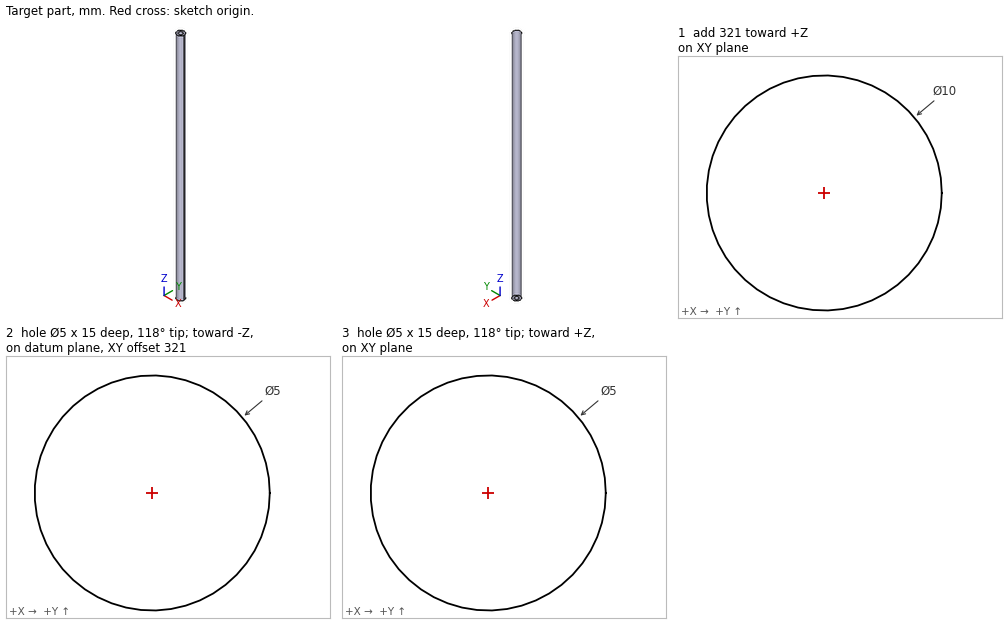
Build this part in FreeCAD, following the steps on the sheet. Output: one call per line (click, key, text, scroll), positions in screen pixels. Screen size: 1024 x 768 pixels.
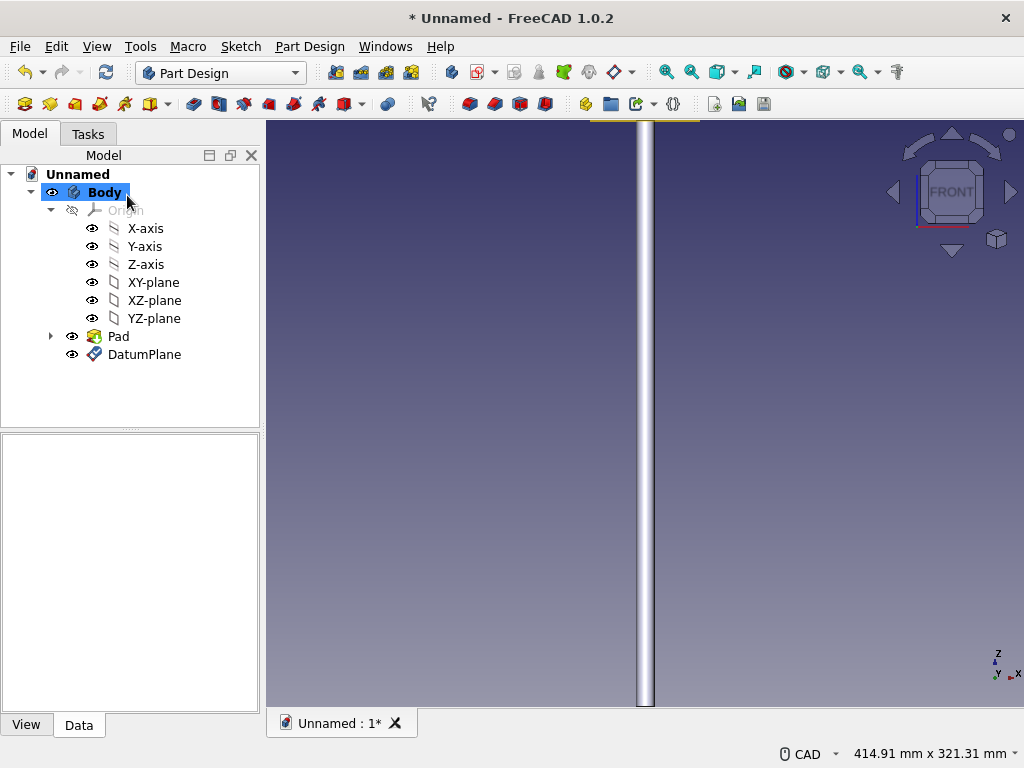
click(117, 354)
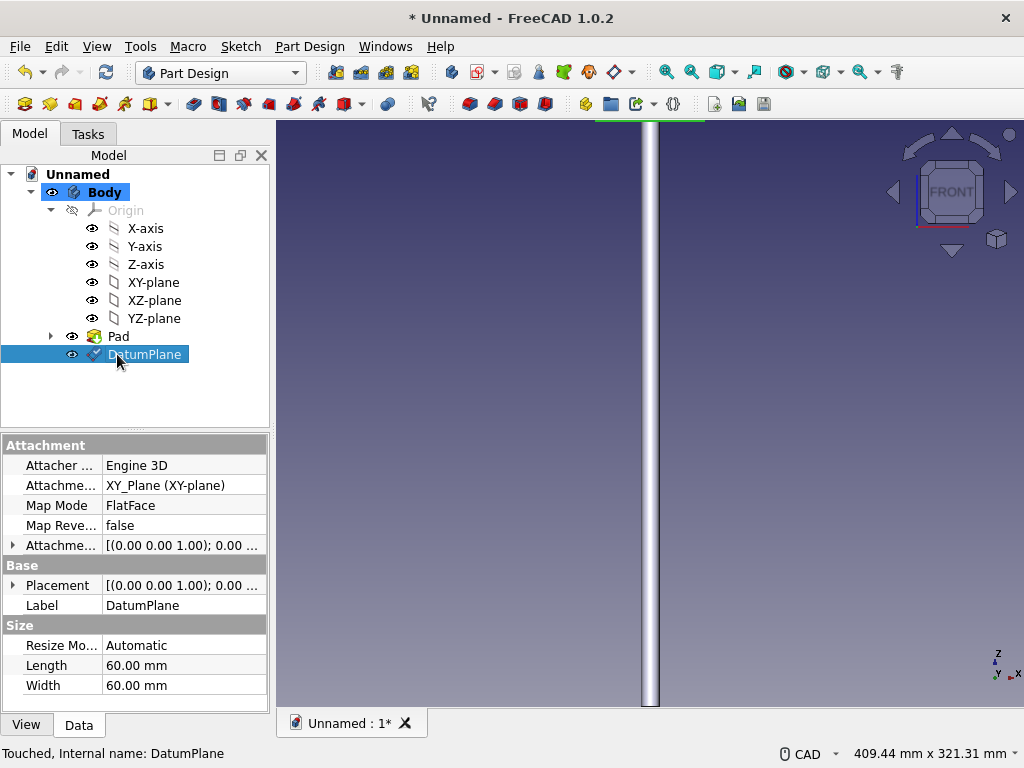
click(476, 72)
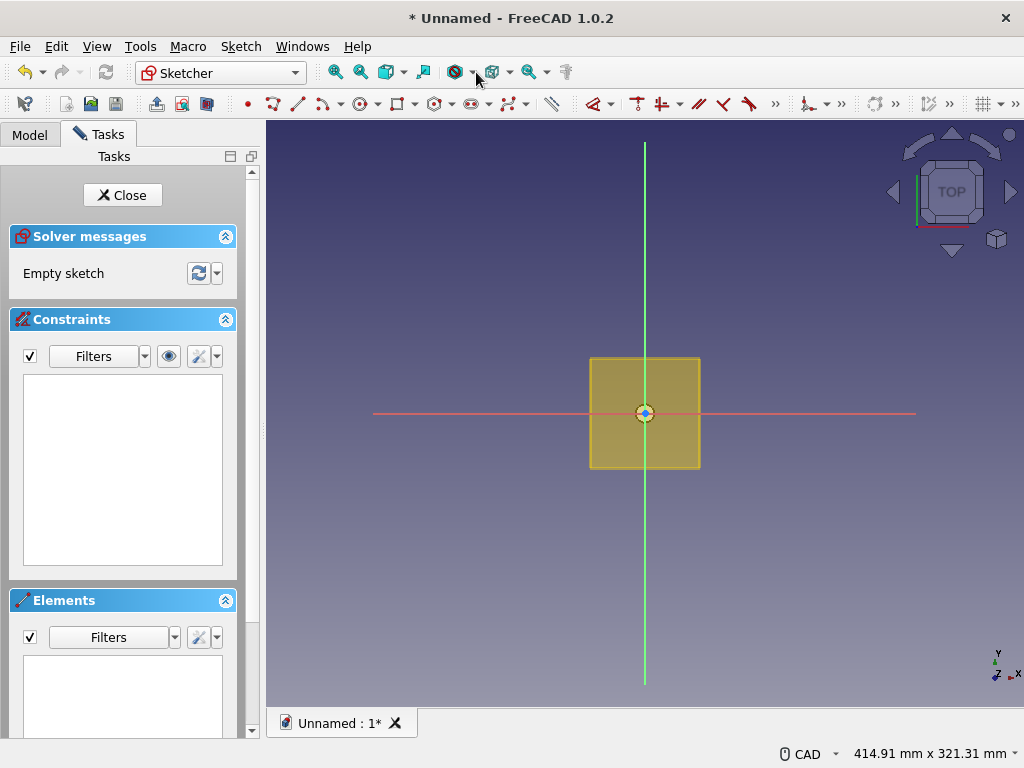
scroll(649, 414, up, 15)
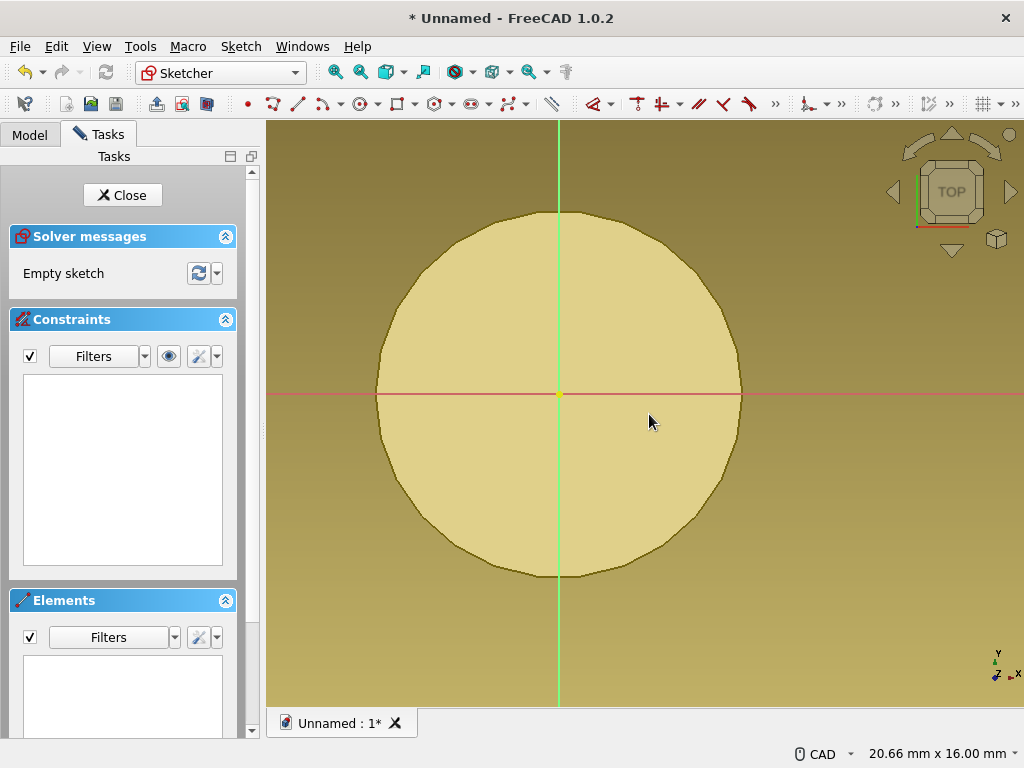
scroll(545, 379, up, 4)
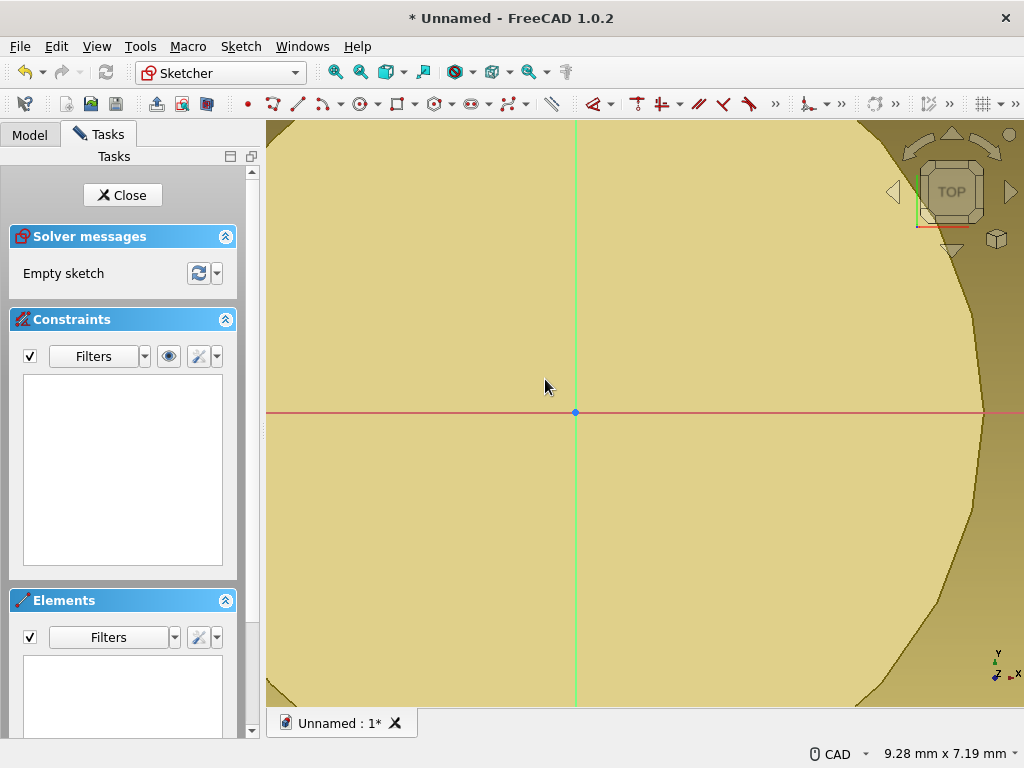
click(360, 104)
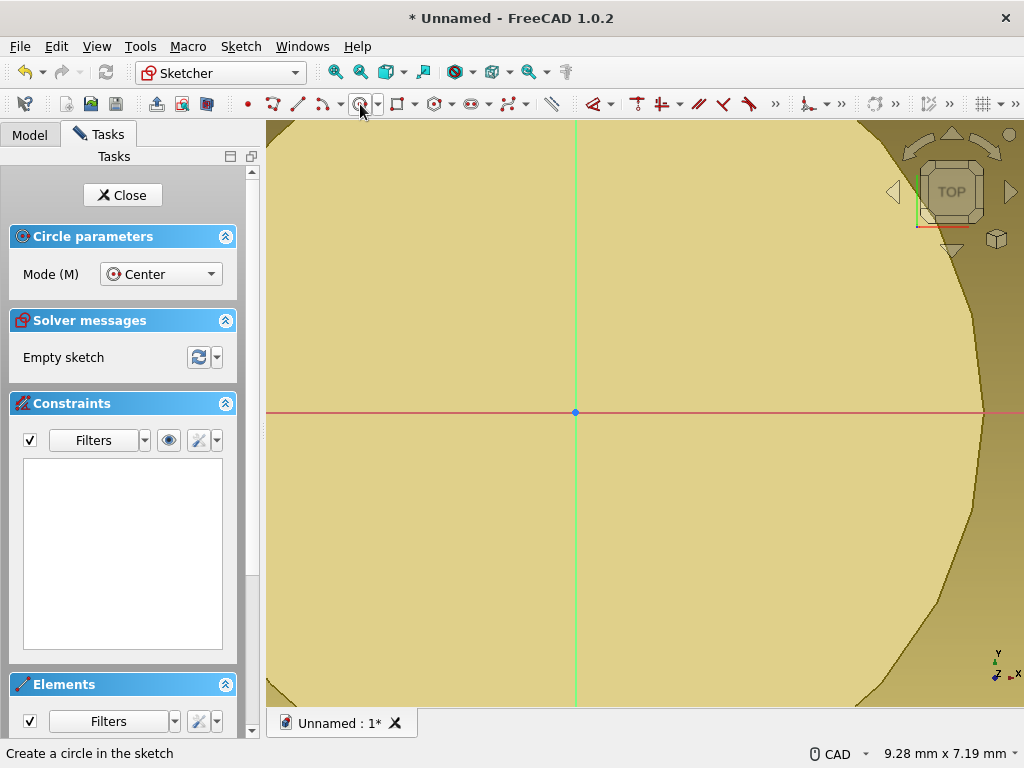
click(576, 413)
move(720, 268)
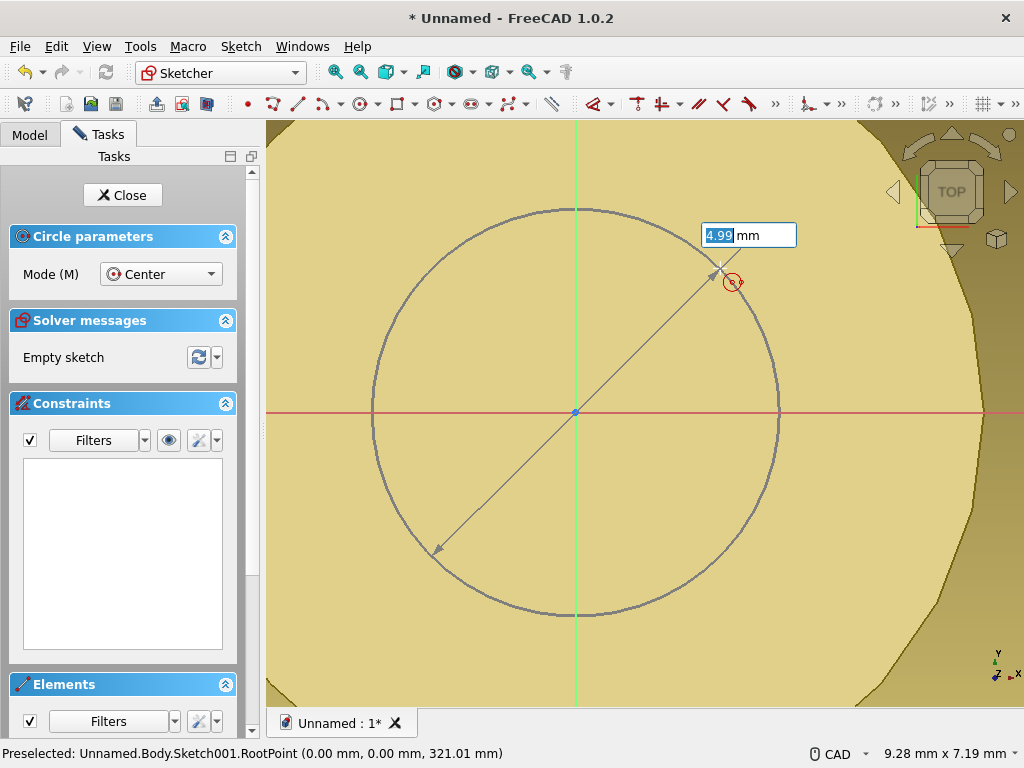
text(5)
key(Return)
key(Escape)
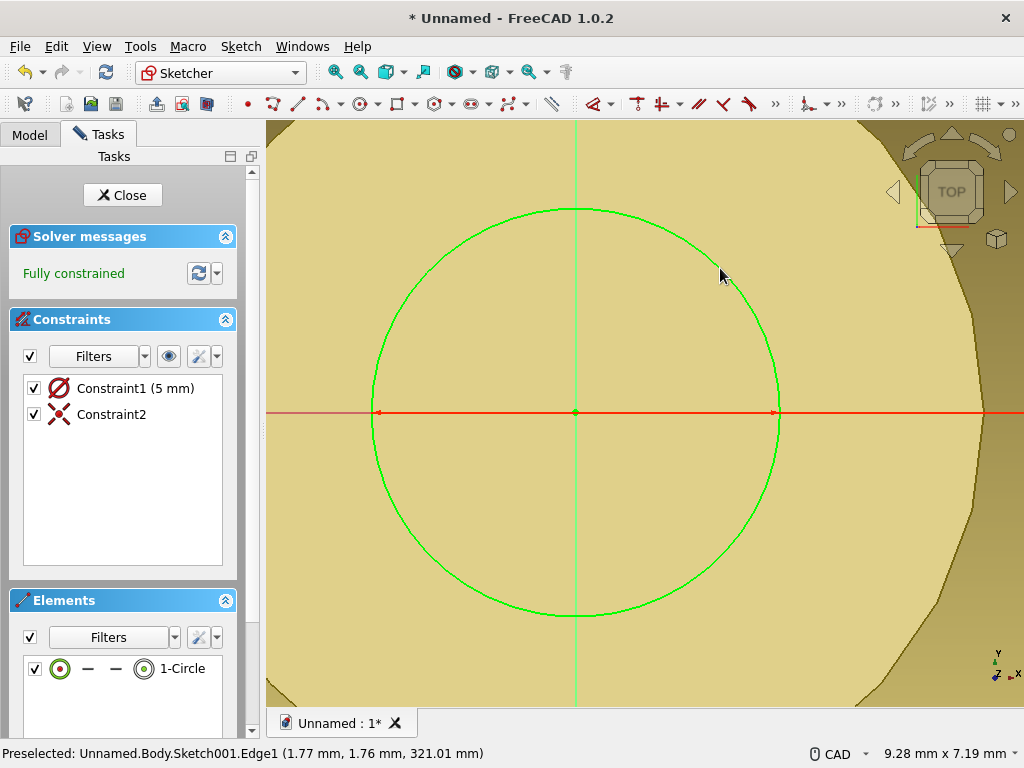
click(123, 195)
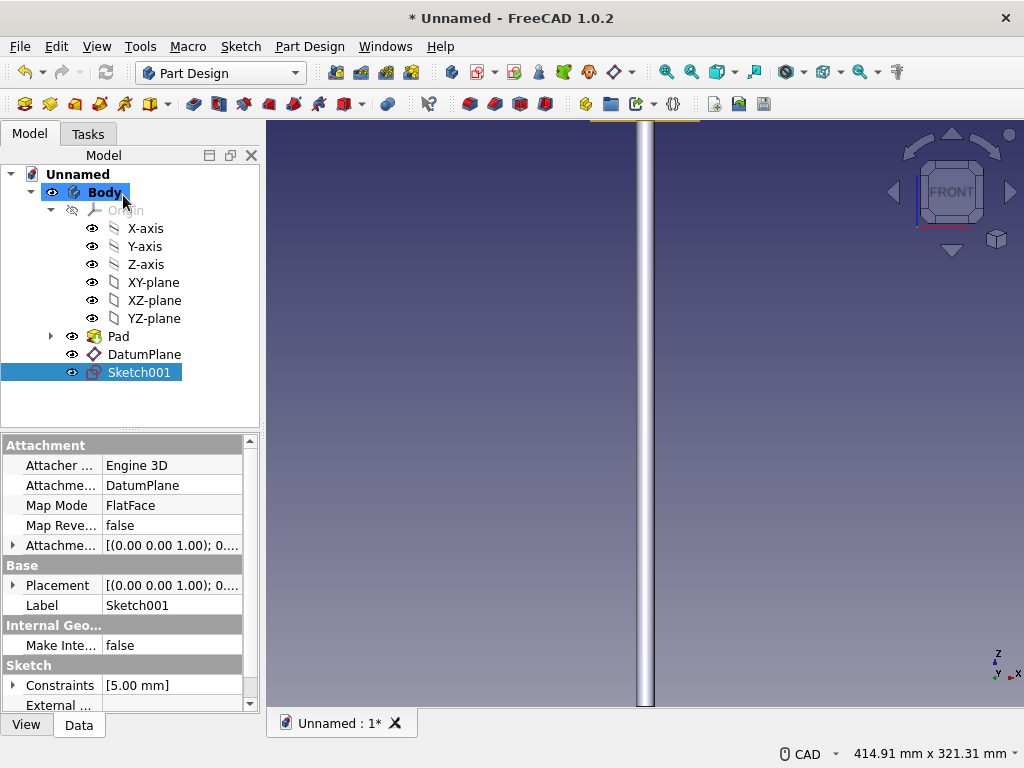
click(219, 104)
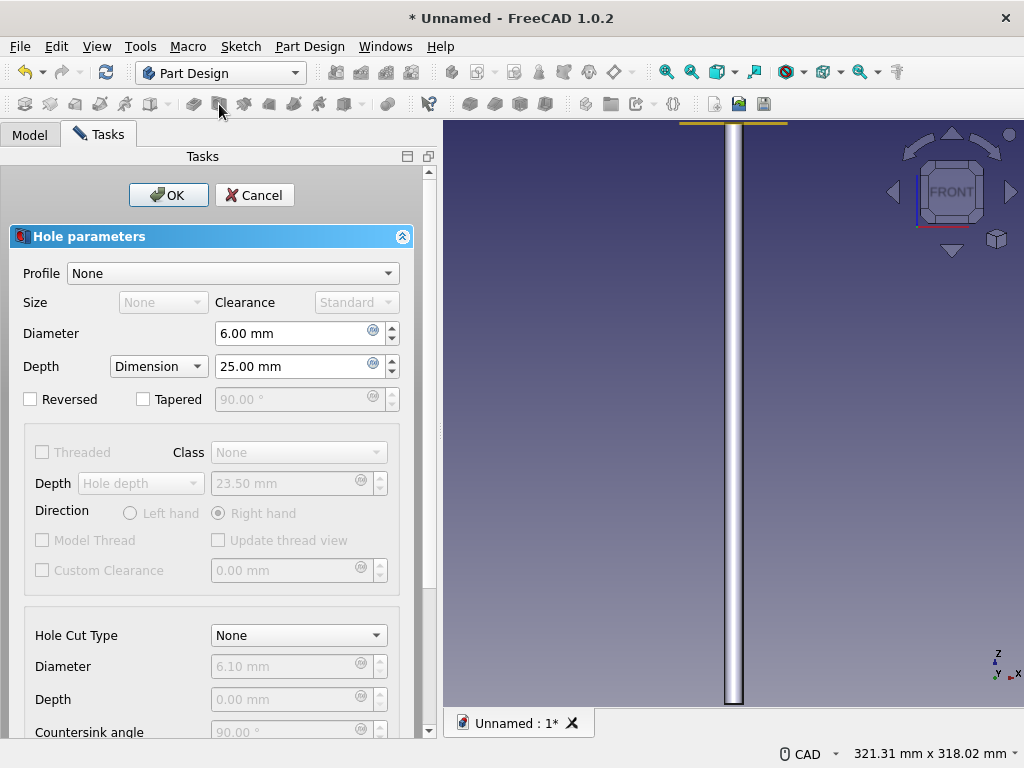
triple_click(300, 334)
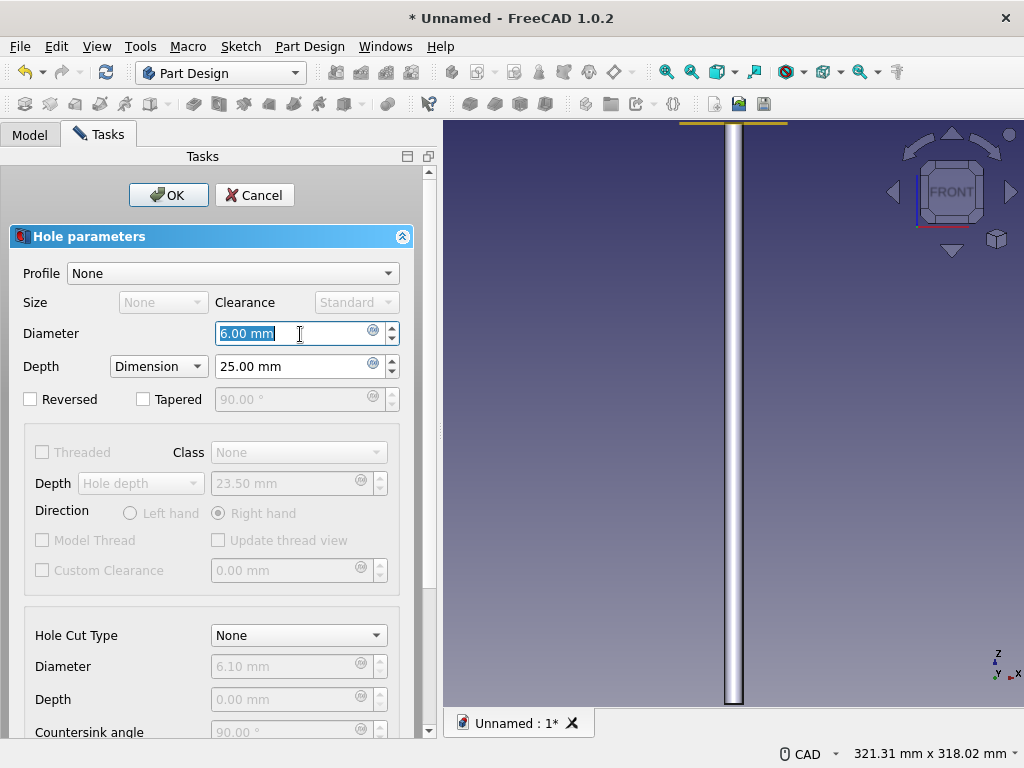
text(5)
key(Tab)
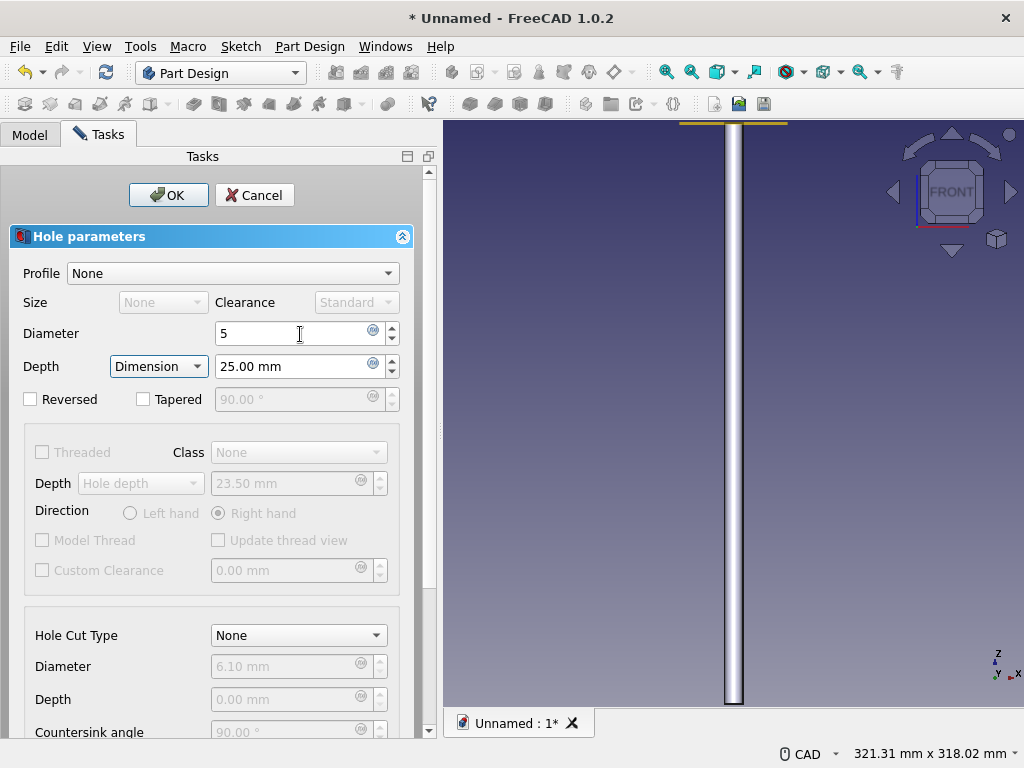
triple_click(300, 366)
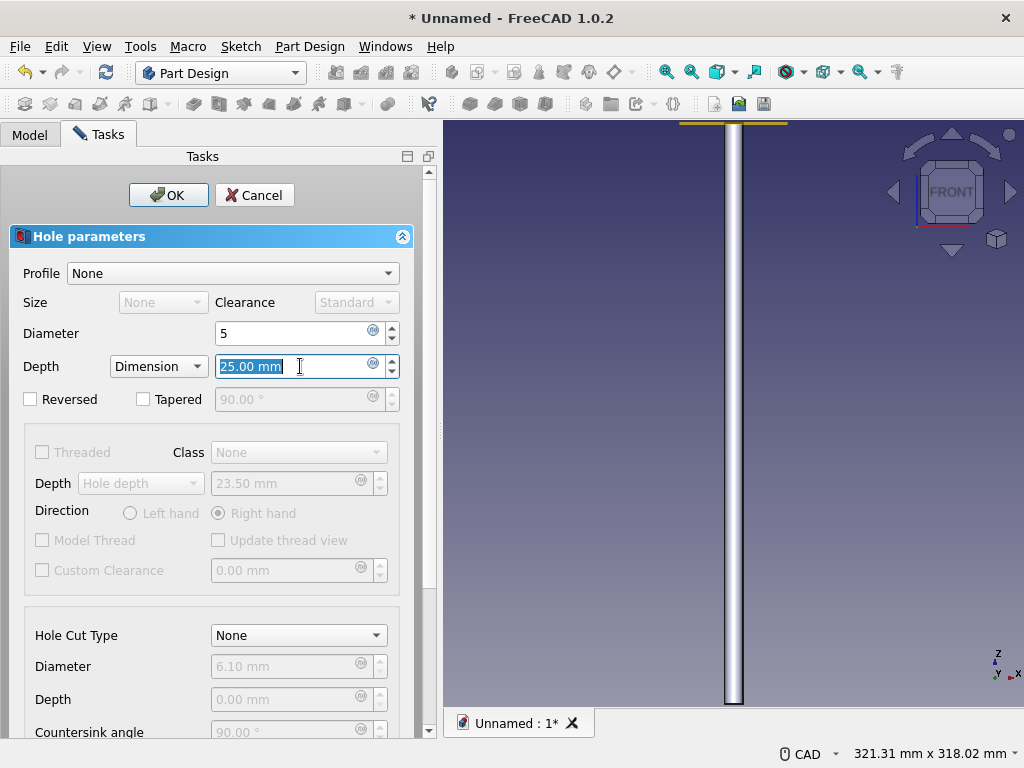
text(15)
key(Tab)